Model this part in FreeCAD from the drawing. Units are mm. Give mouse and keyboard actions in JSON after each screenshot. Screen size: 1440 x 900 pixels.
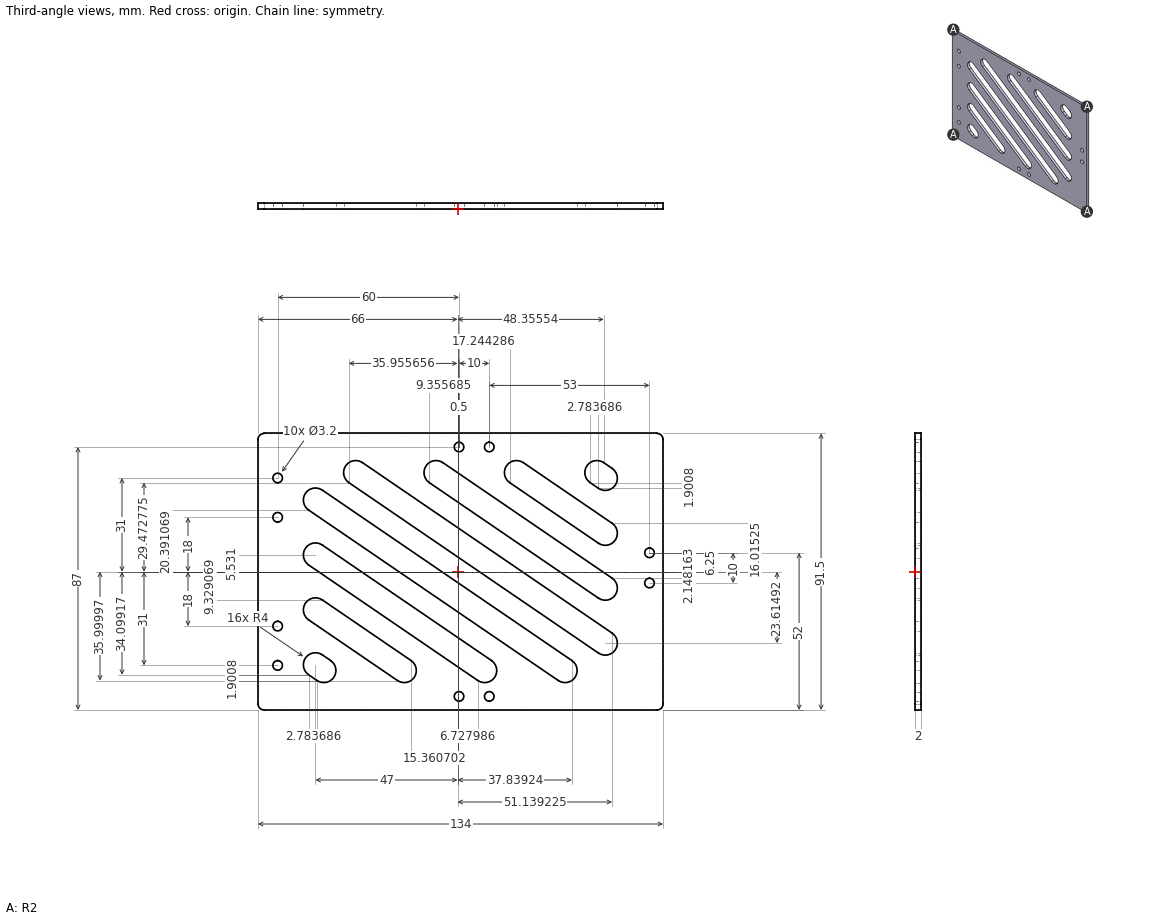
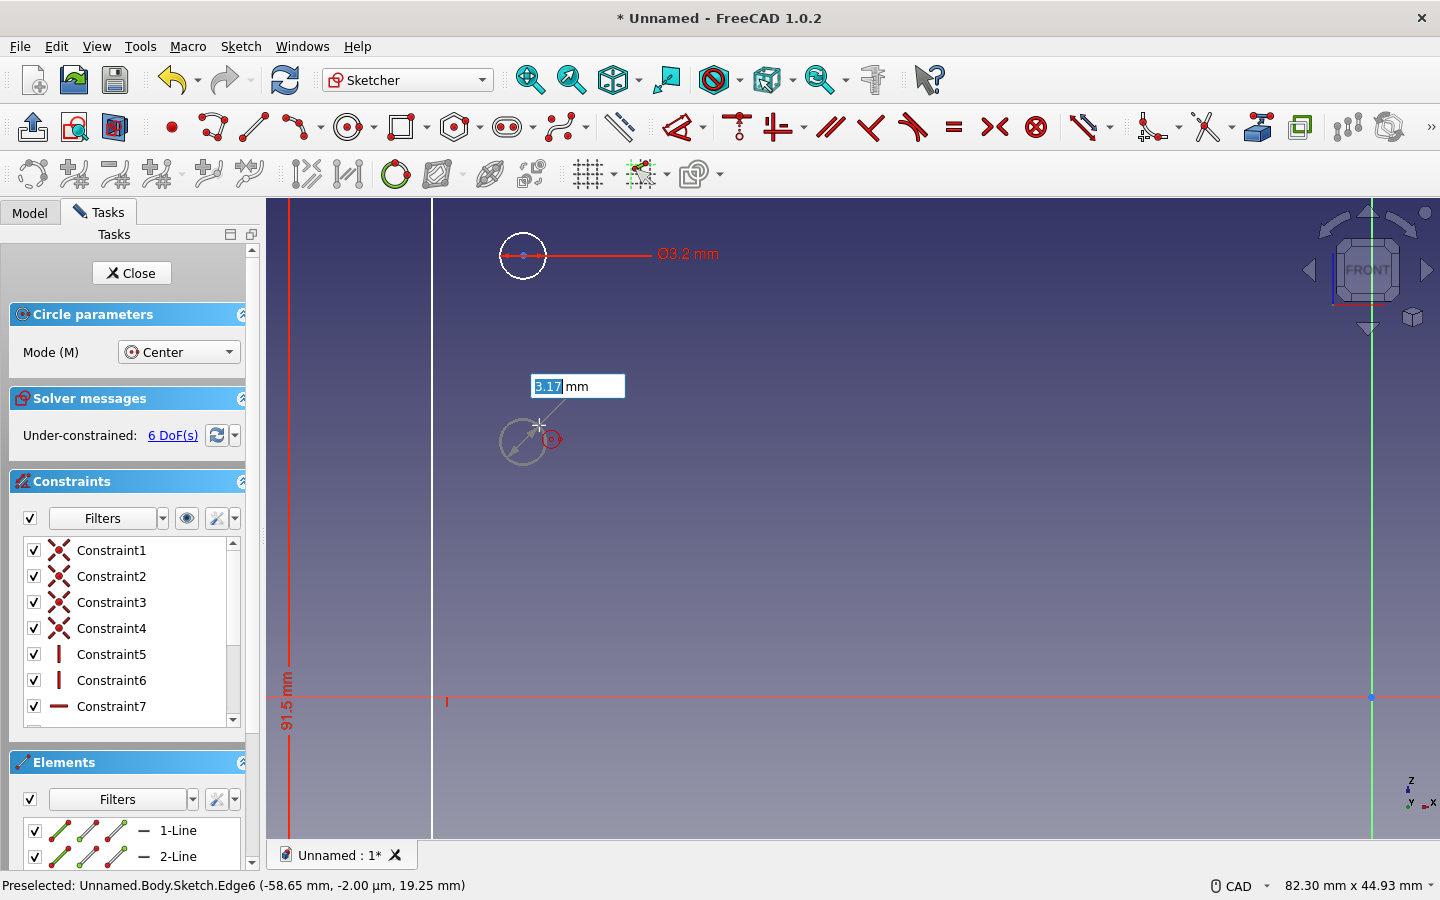
{"action": "type", "text": "3.2"}
{"action": "key", "text": "Return"}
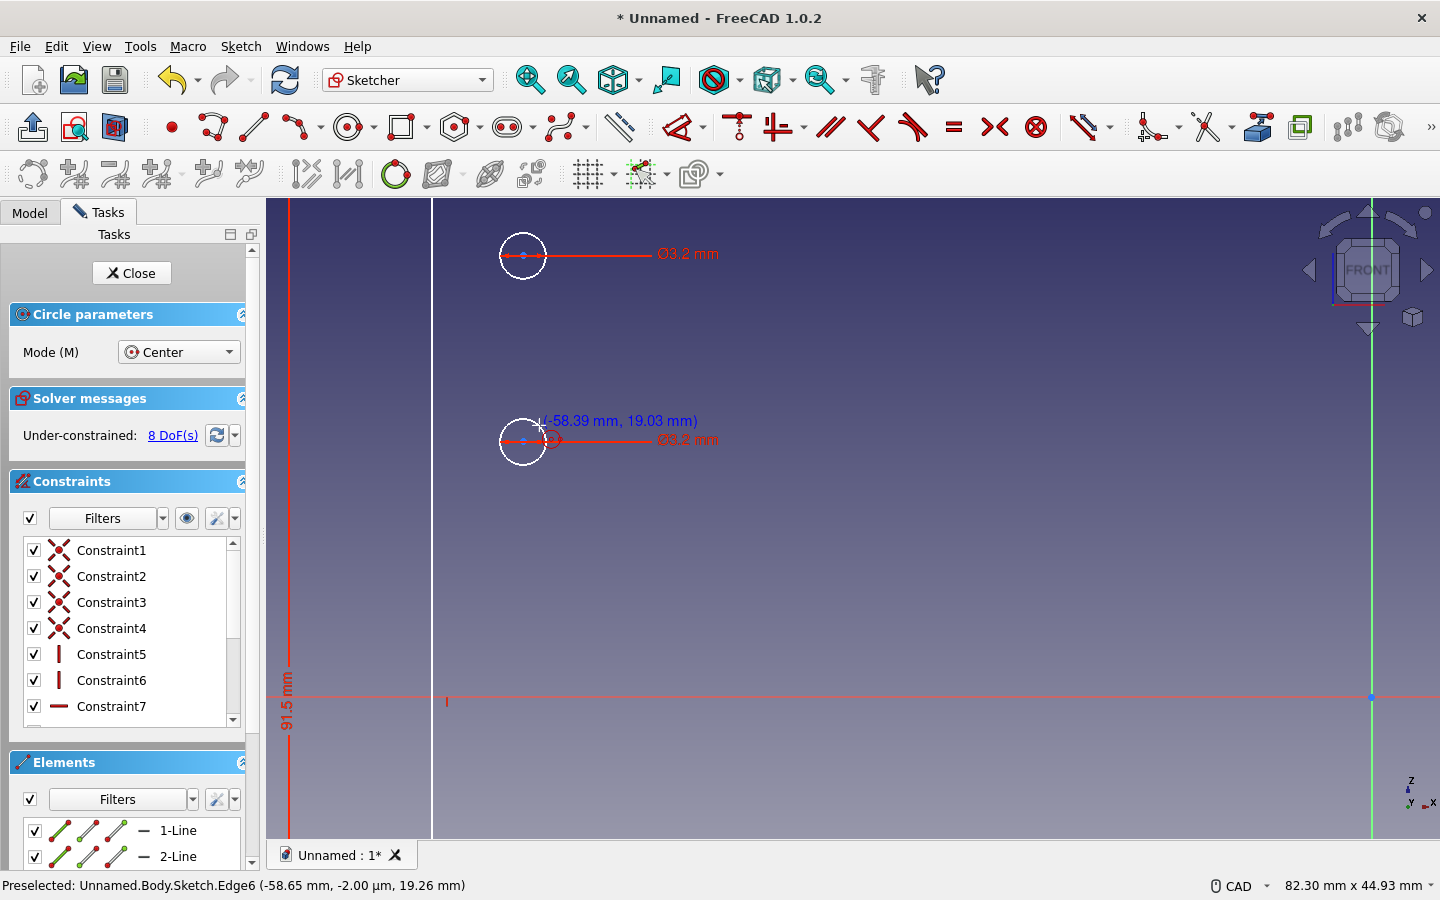
{"action": "scroll", "coordinate": [525, 441], "scroll_direction": "down", "scroll_amount": 6}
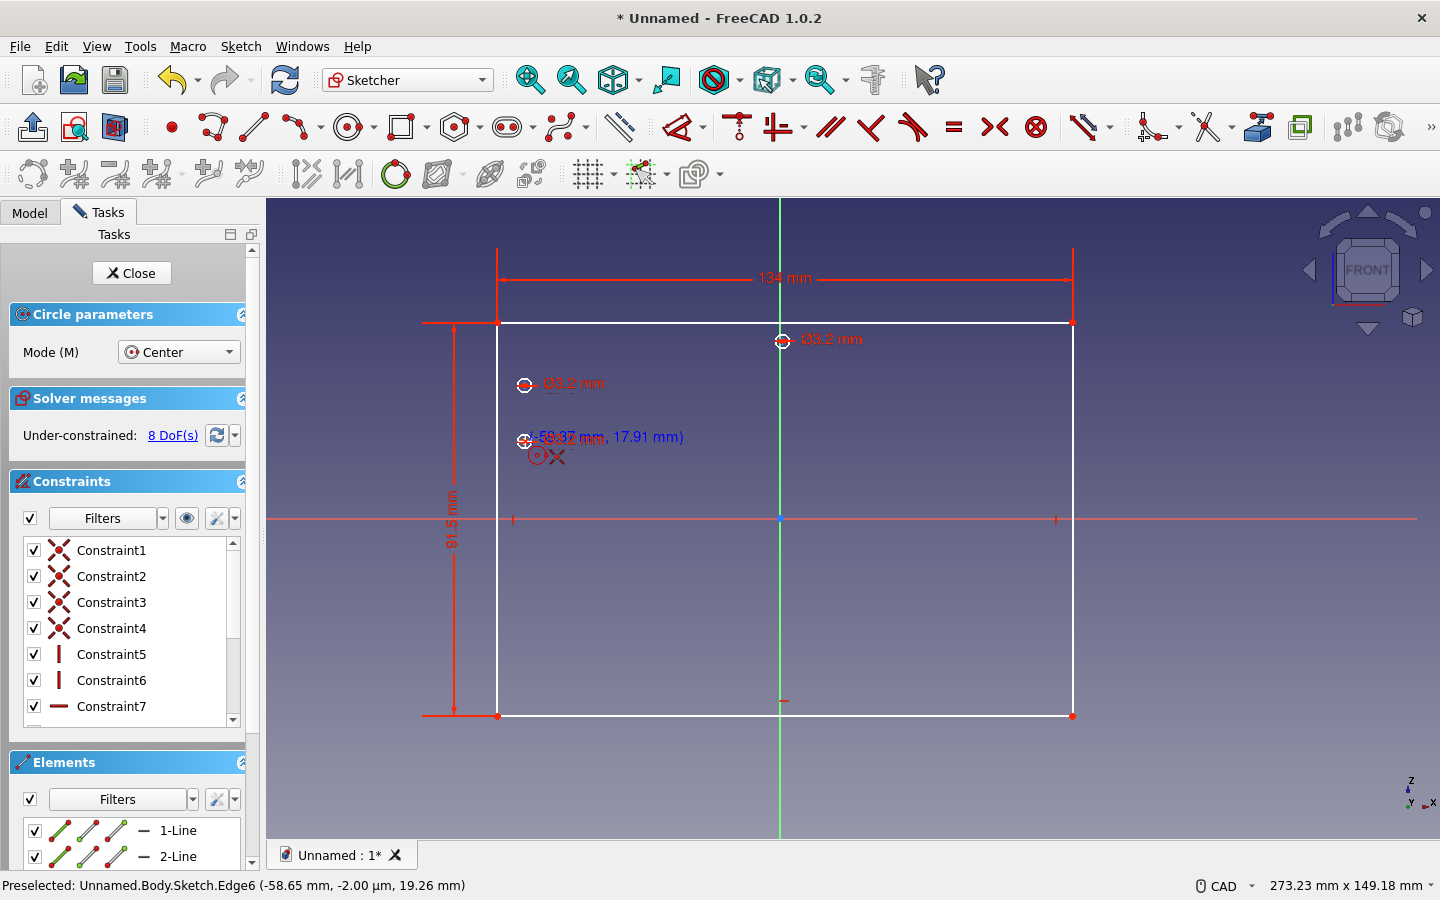
{"action": "scroll", "coordinate": [825, 341], "scroll_direction": "up", "scroll_amount": 6}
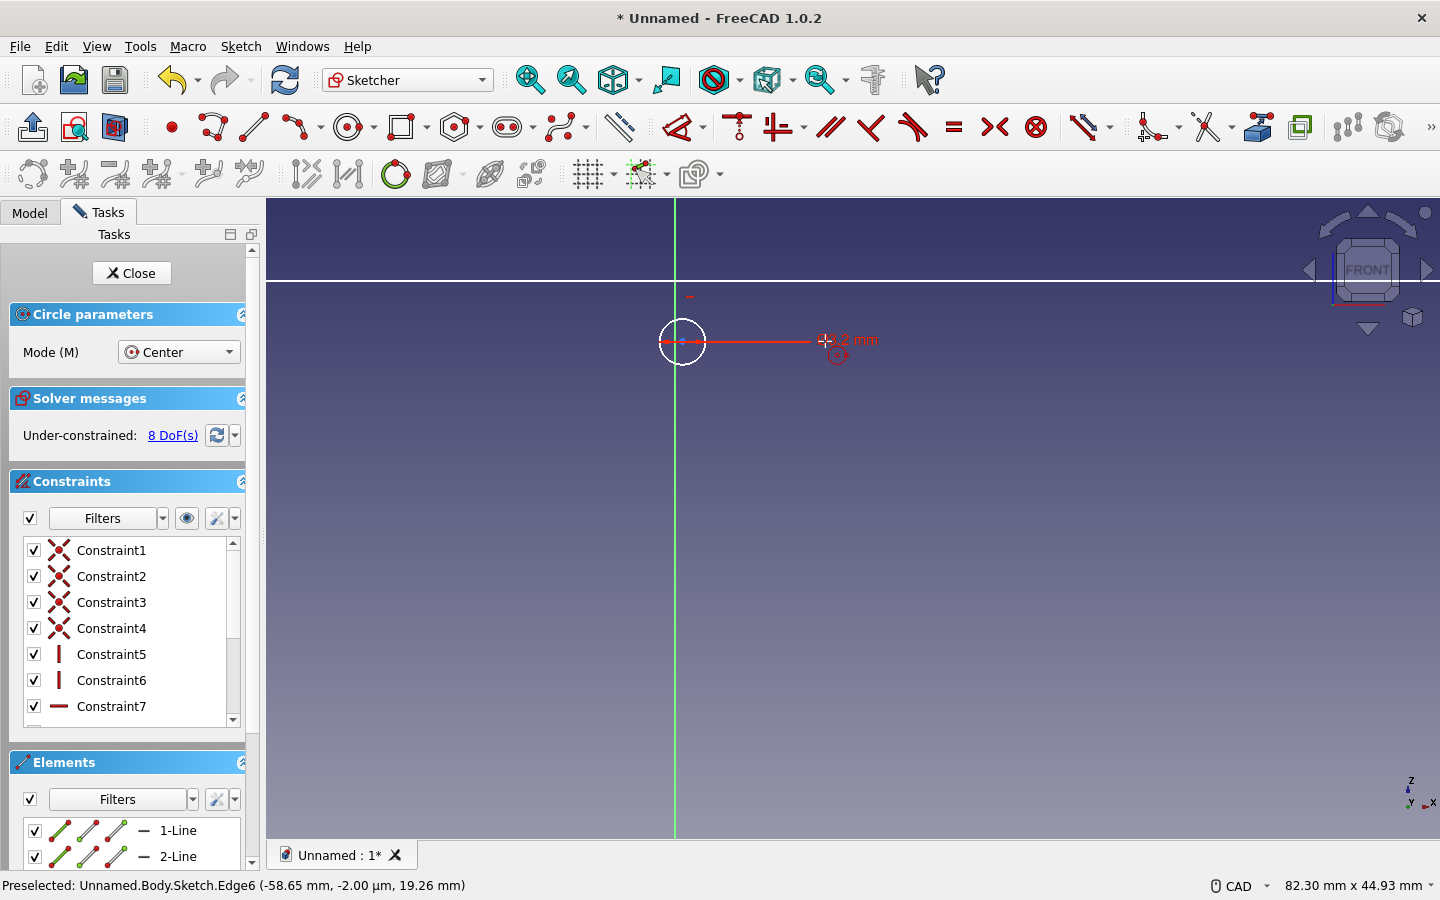
{"action": "left_click", "coordinate": [825, 341]}
{"action": "mouse_move", "coordinate": [841, 325]}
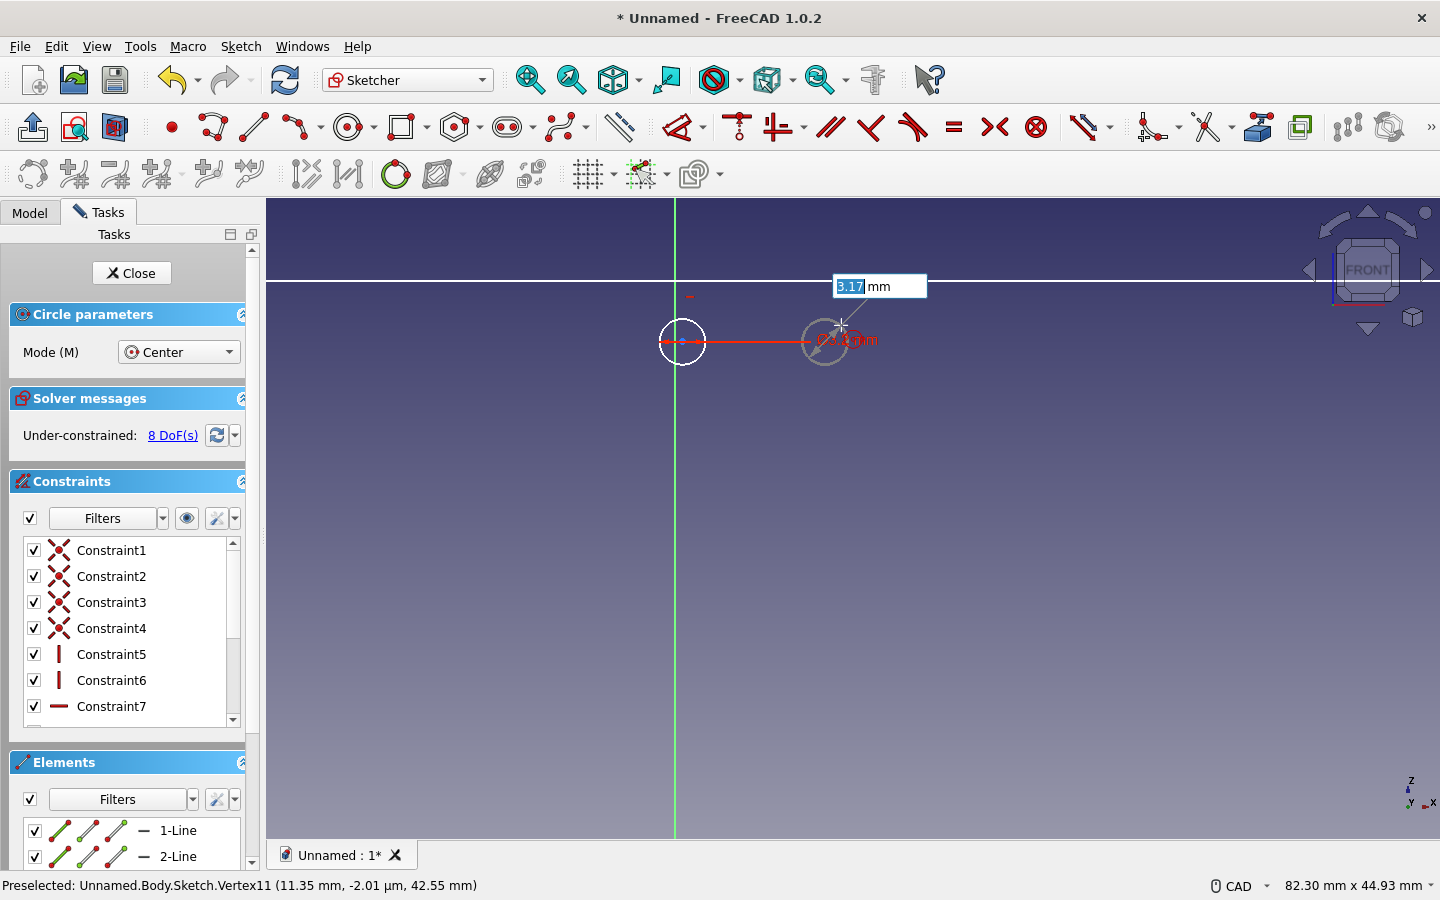
{"action": "type", "text": "3.2"}
{"action": "key", "text": "Return"}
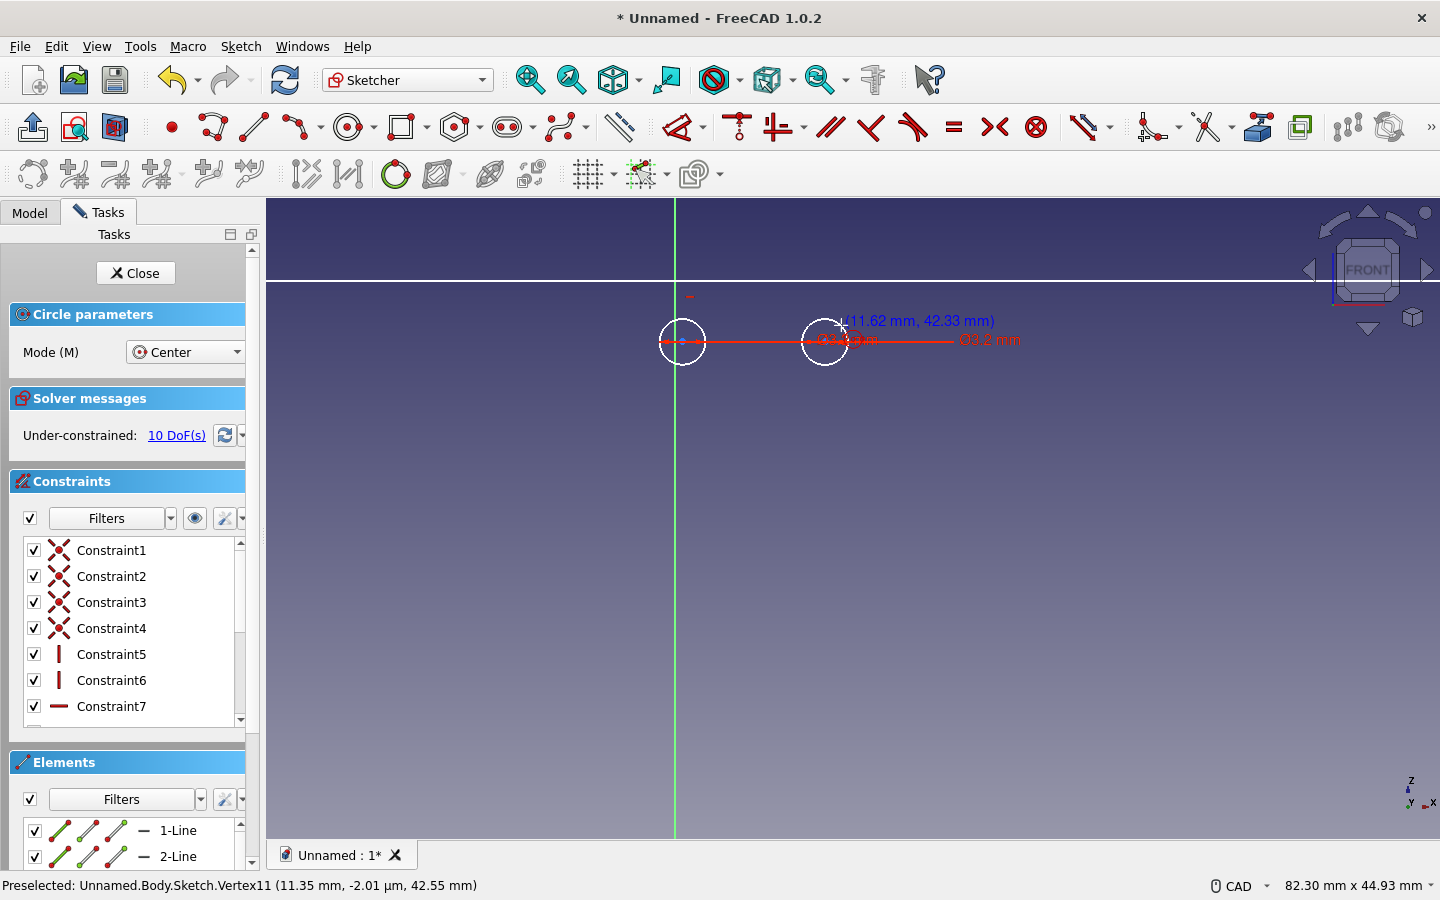
{"action": "scroll", "coordinate": [825, 341], "scroll_direction": "down", "scroll_amount": 6}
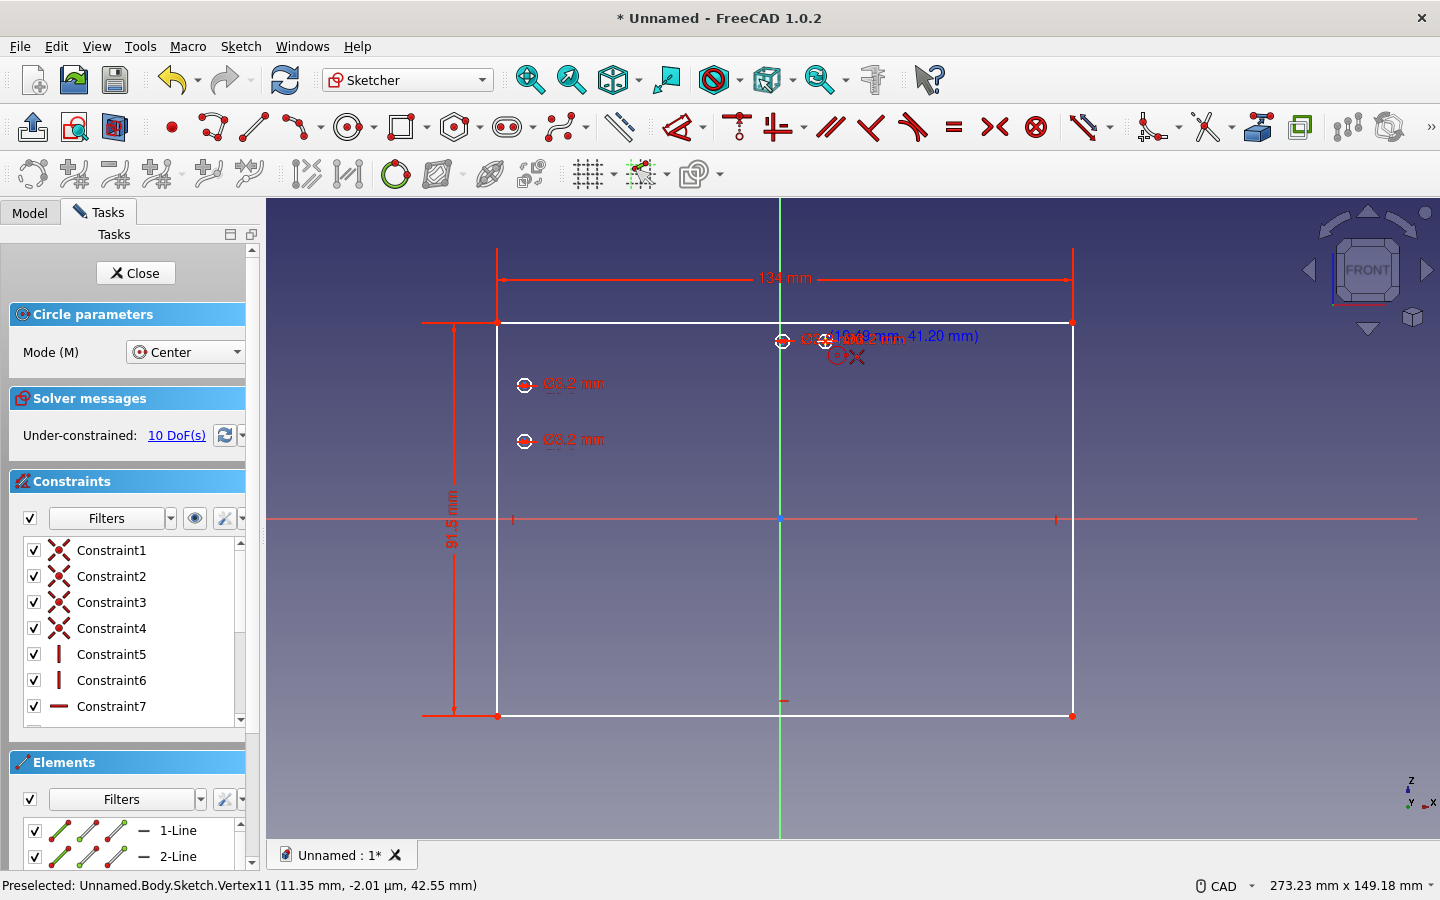
{"action": "scroll", "coordinate": [1053, 492], "scroll_direction": "up", "scroll_amount": 6}